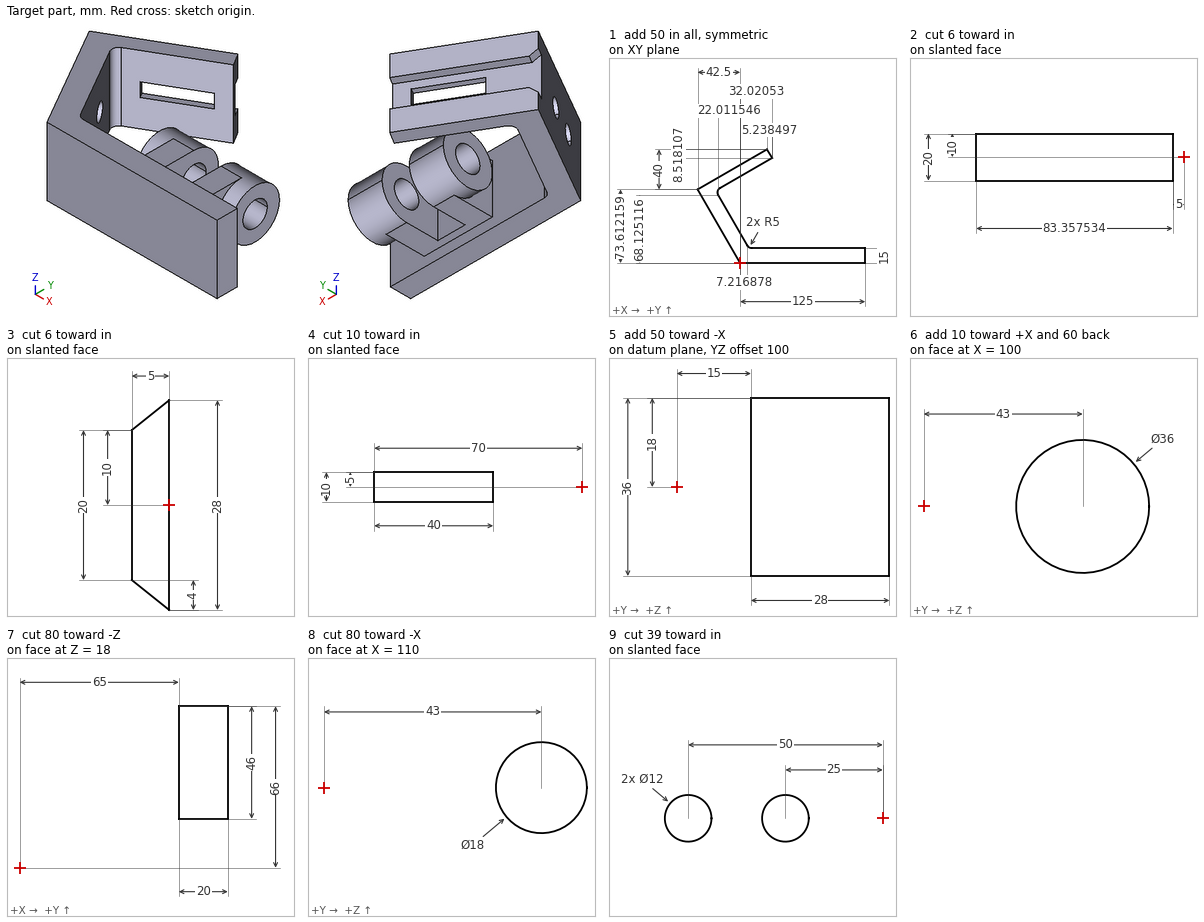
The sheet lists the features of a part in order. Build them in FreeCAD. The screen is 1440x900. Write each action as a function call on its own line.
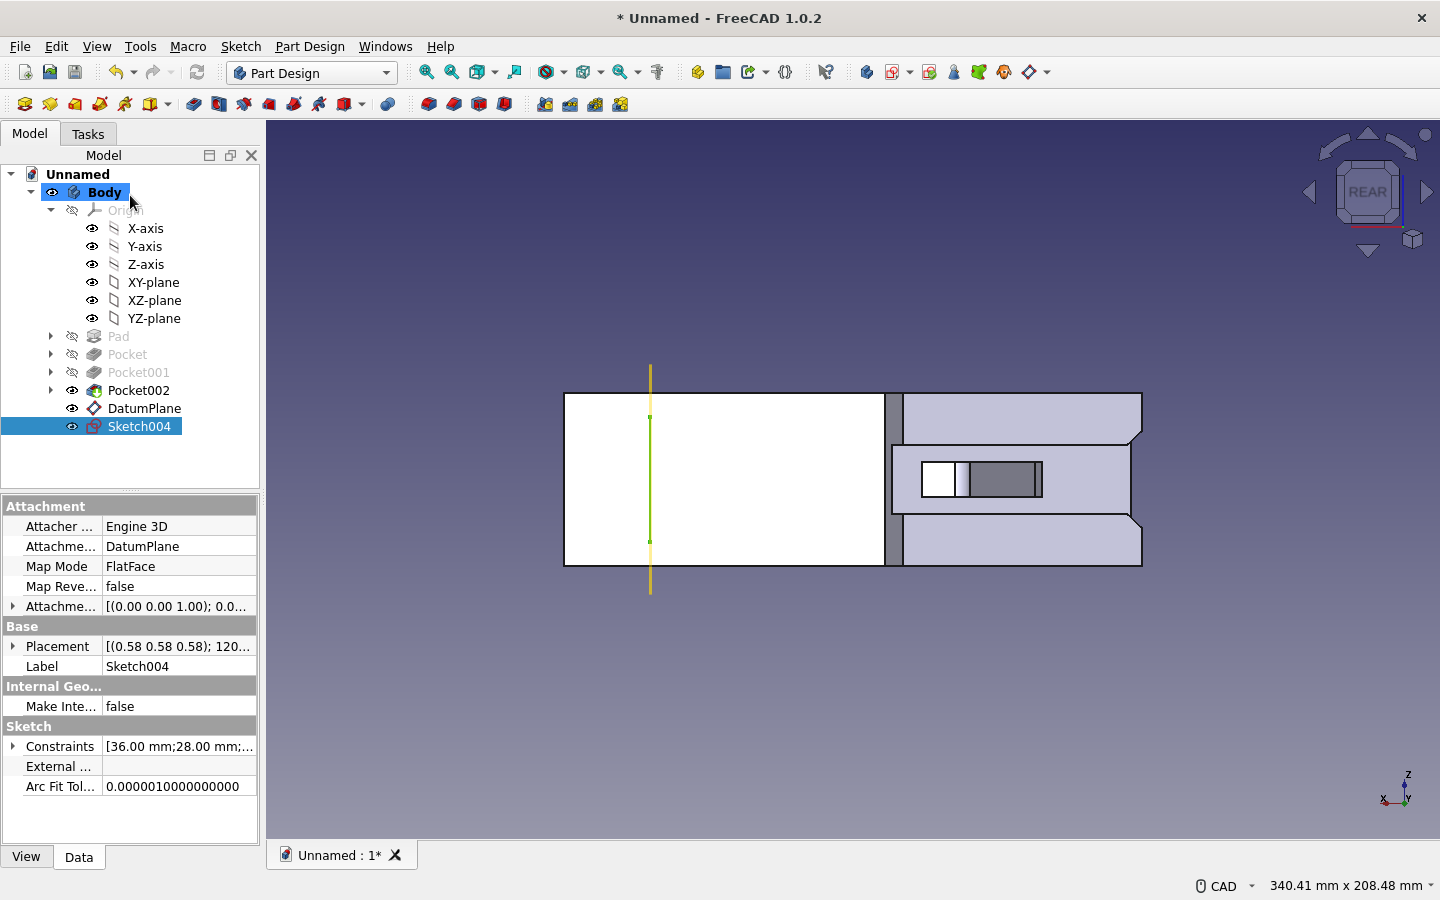
click(25, 104)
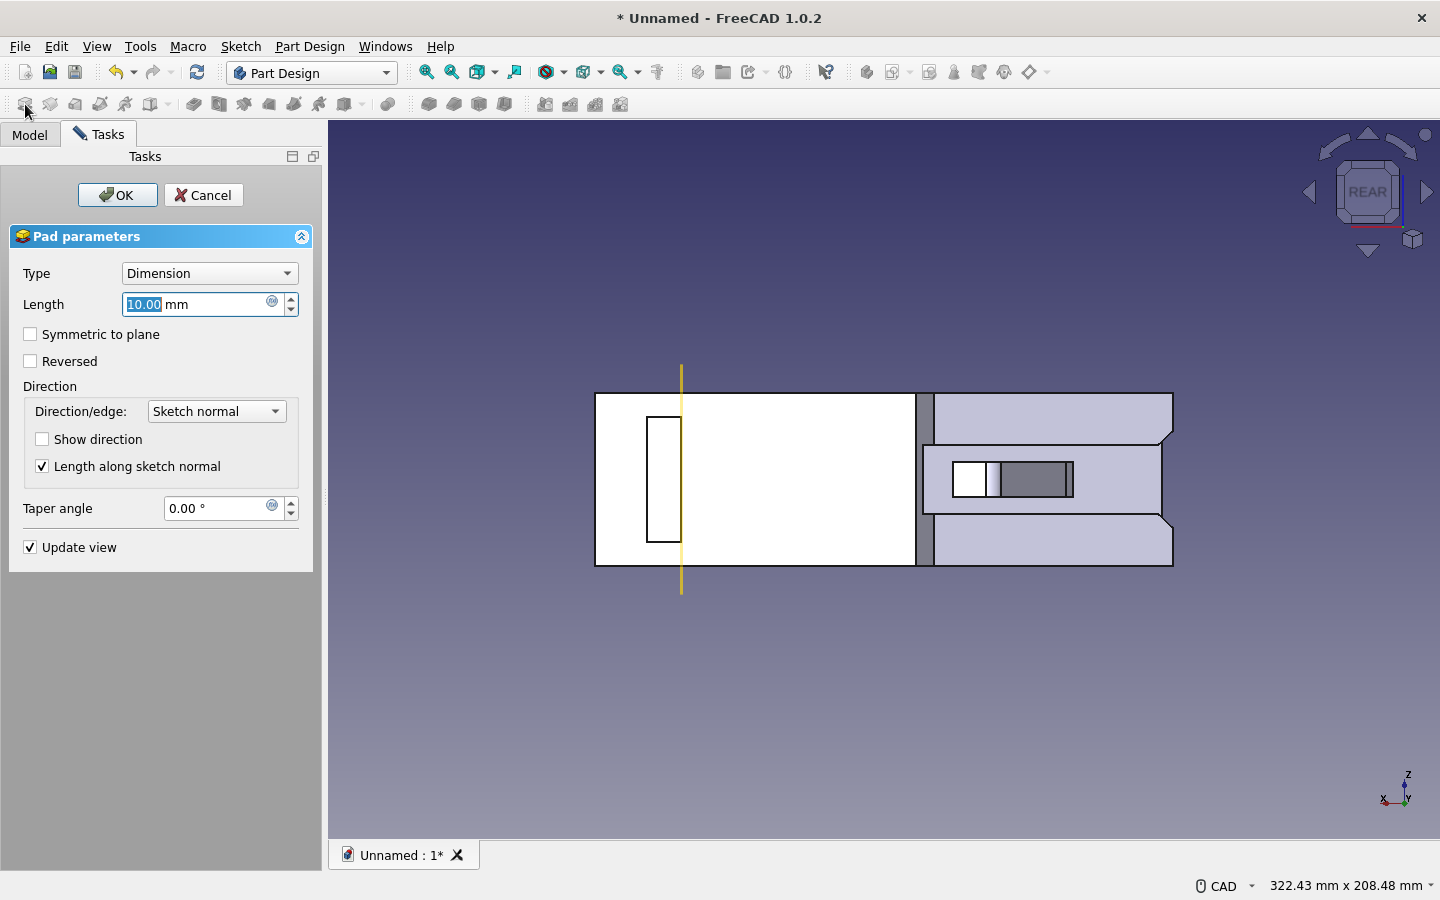
text(50)
key(Tab)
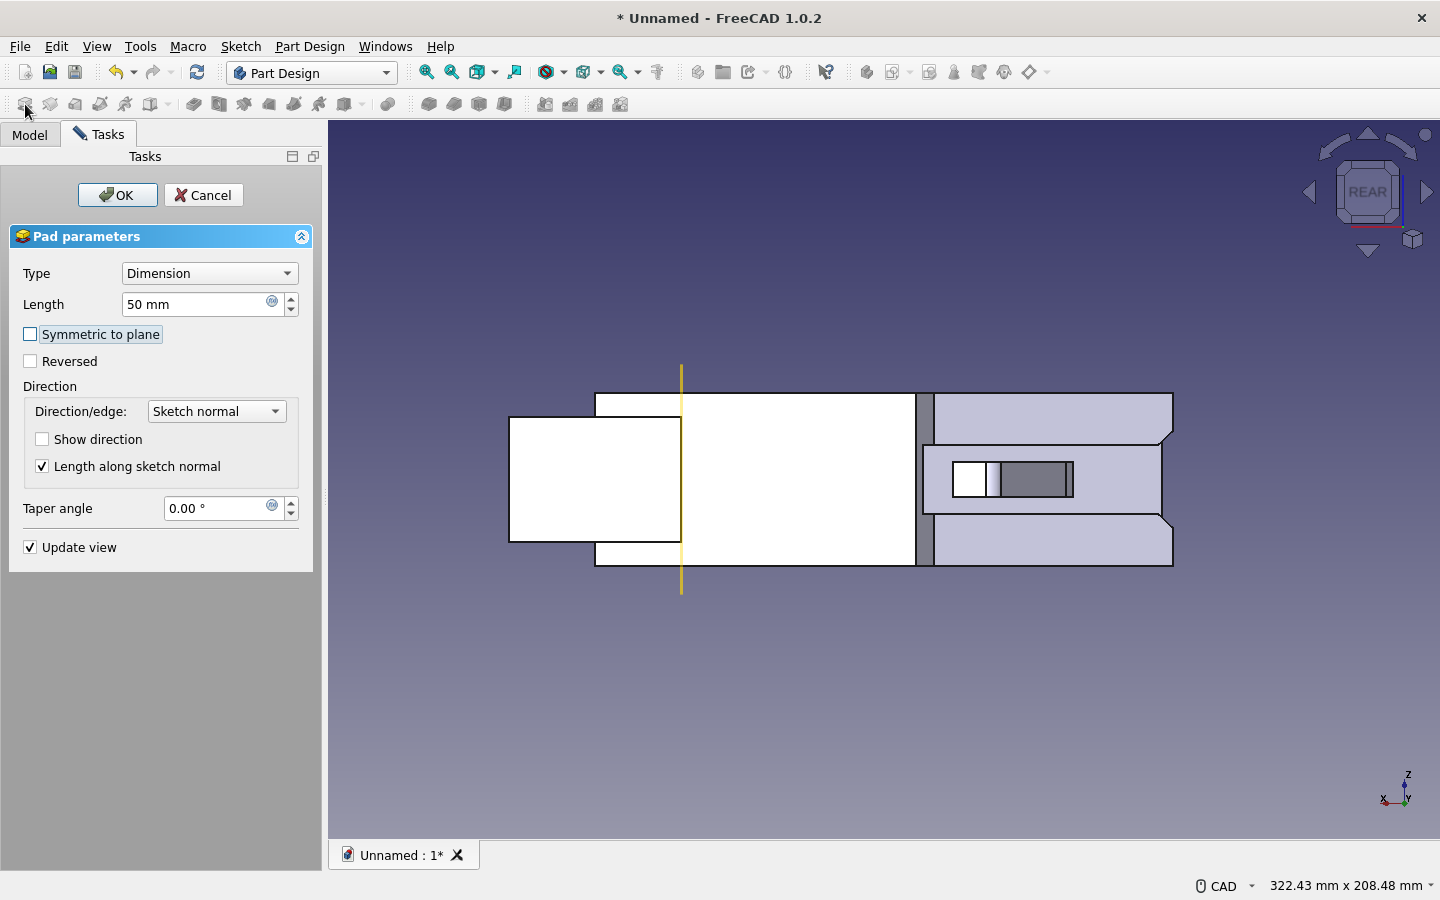
click(31, 361)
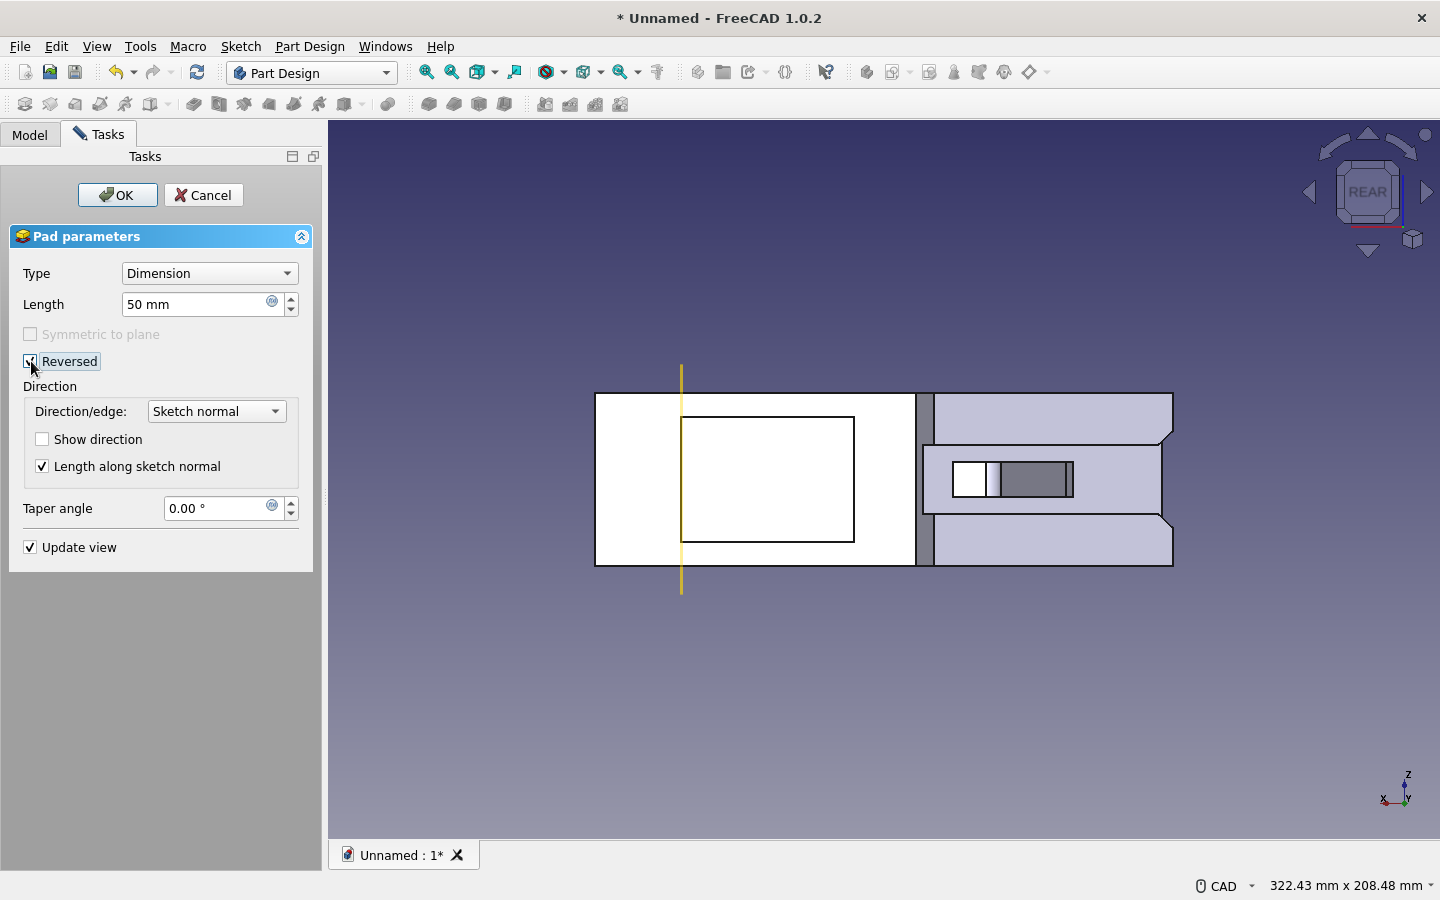
click(118, 195)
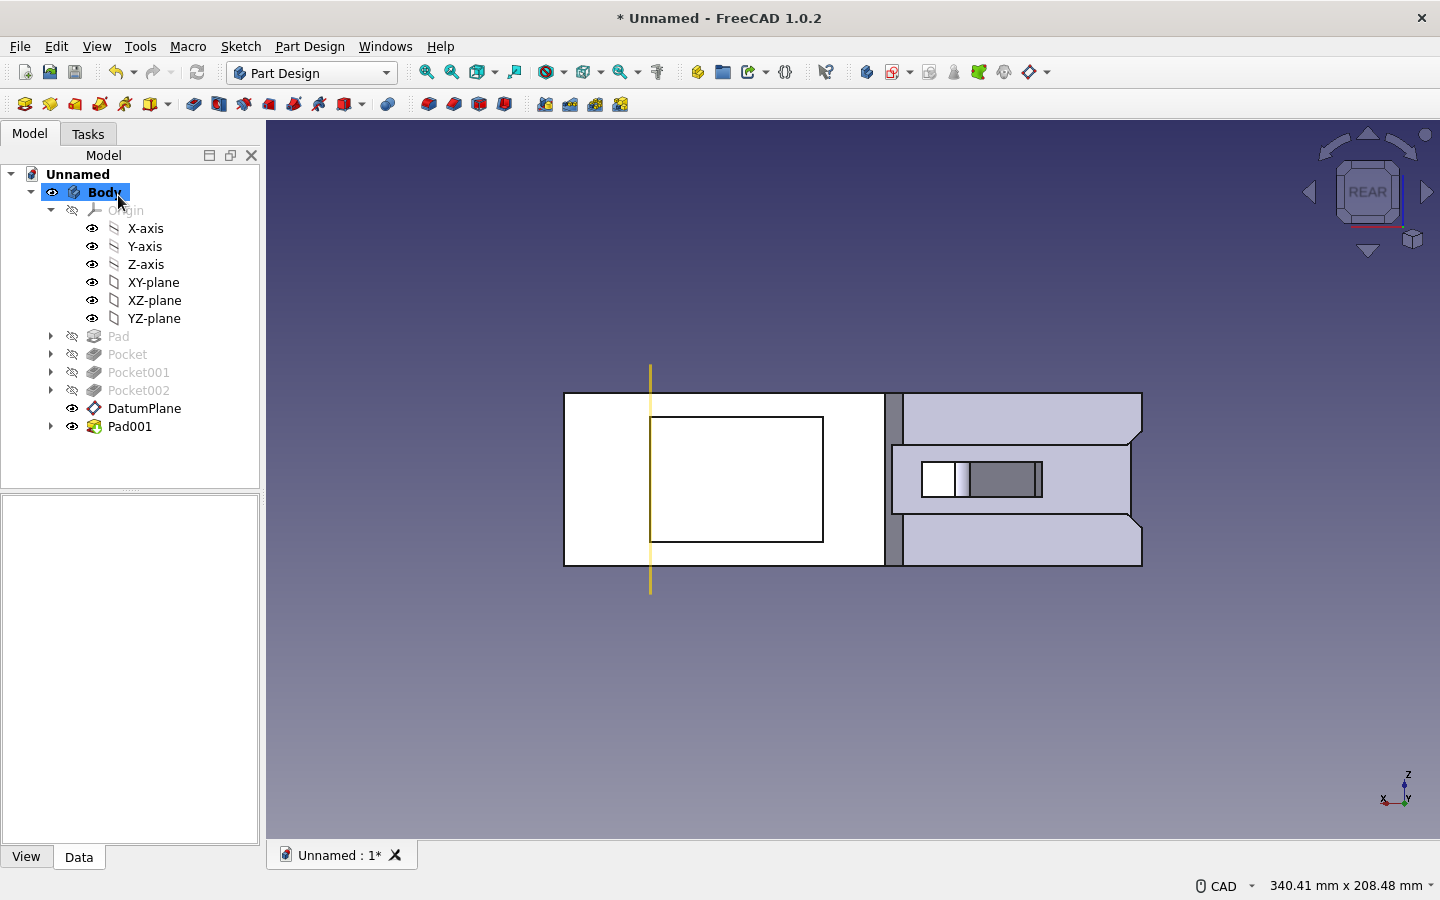
click(117, 408)
key(space)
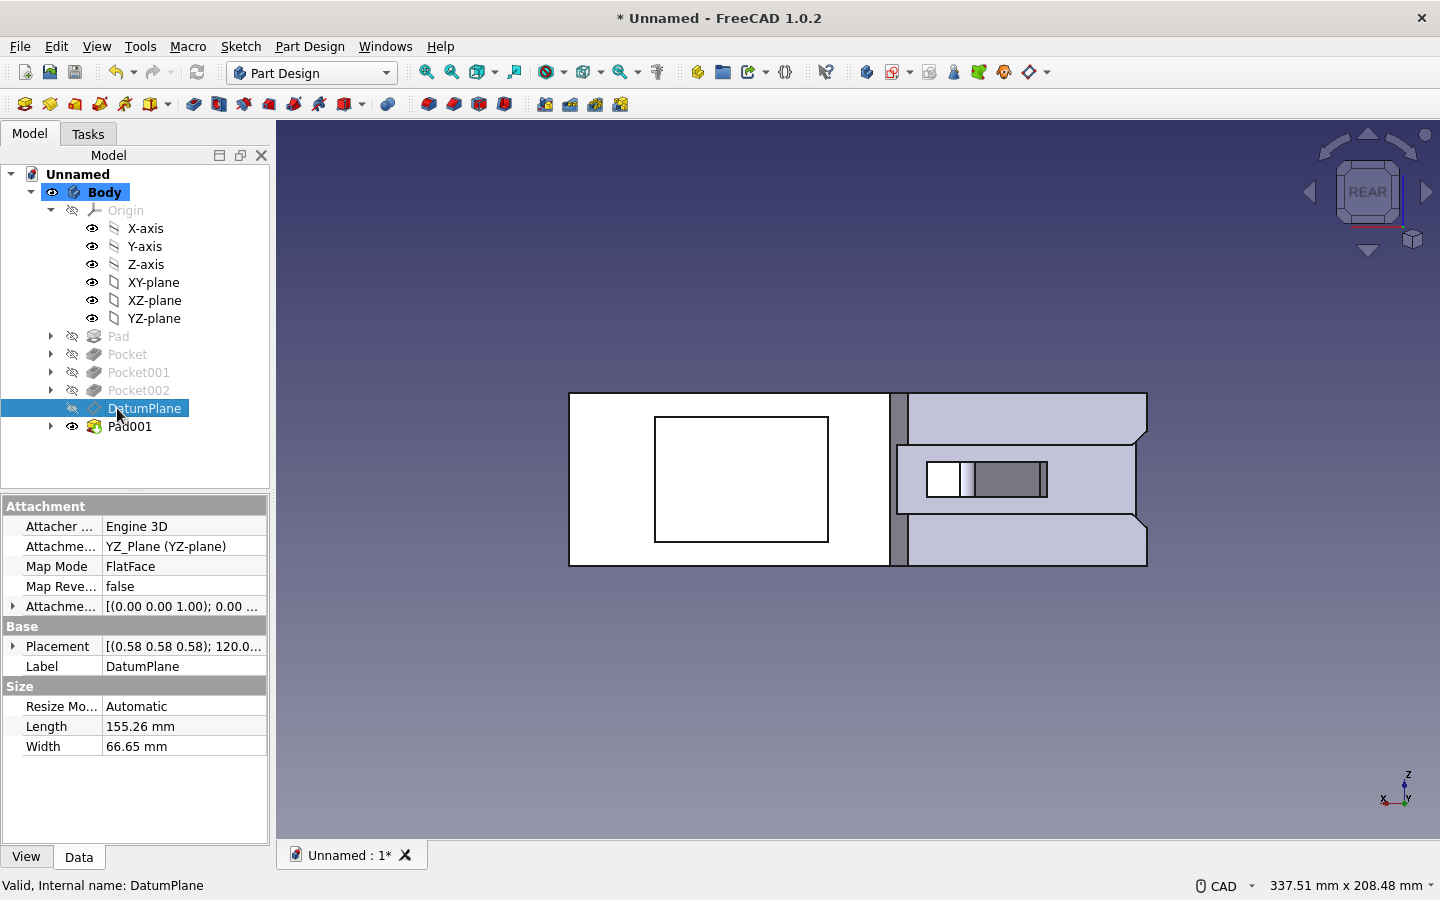
key(0)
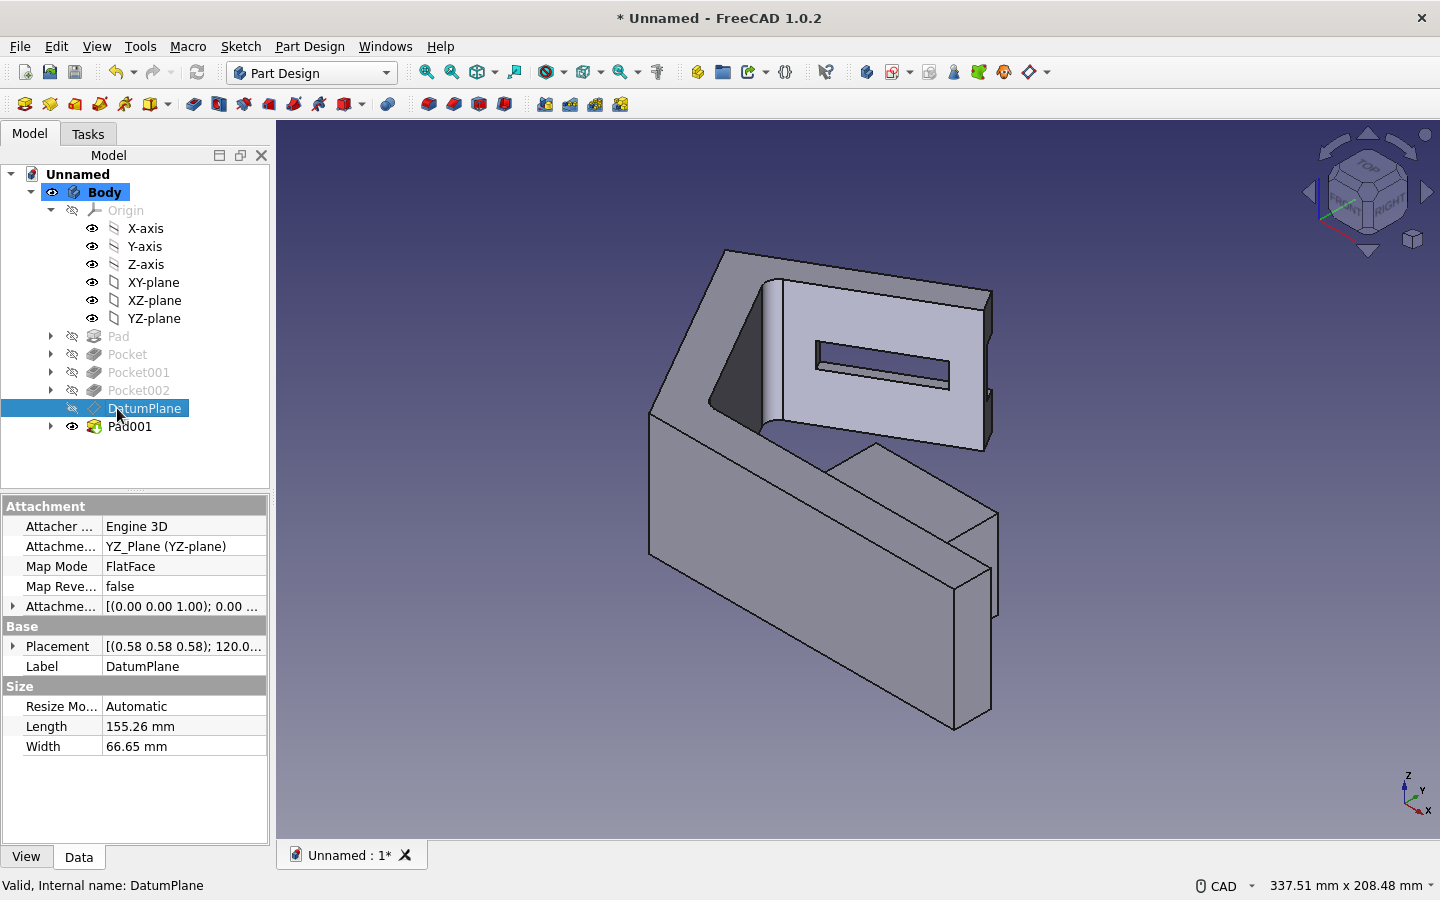
key(3)